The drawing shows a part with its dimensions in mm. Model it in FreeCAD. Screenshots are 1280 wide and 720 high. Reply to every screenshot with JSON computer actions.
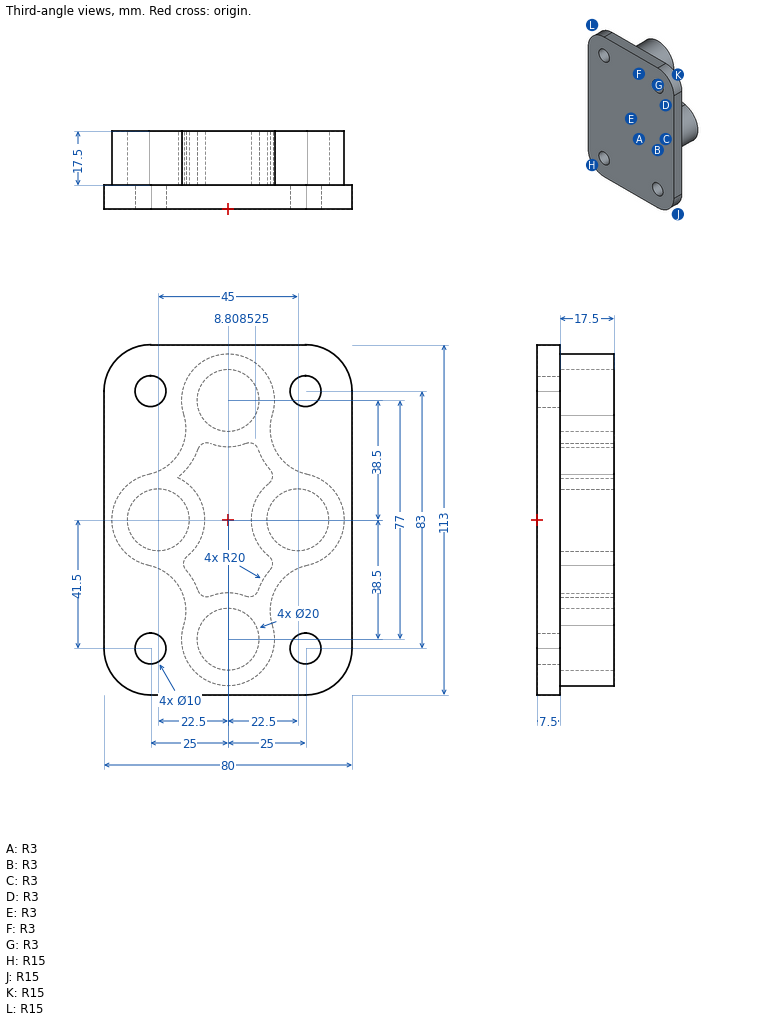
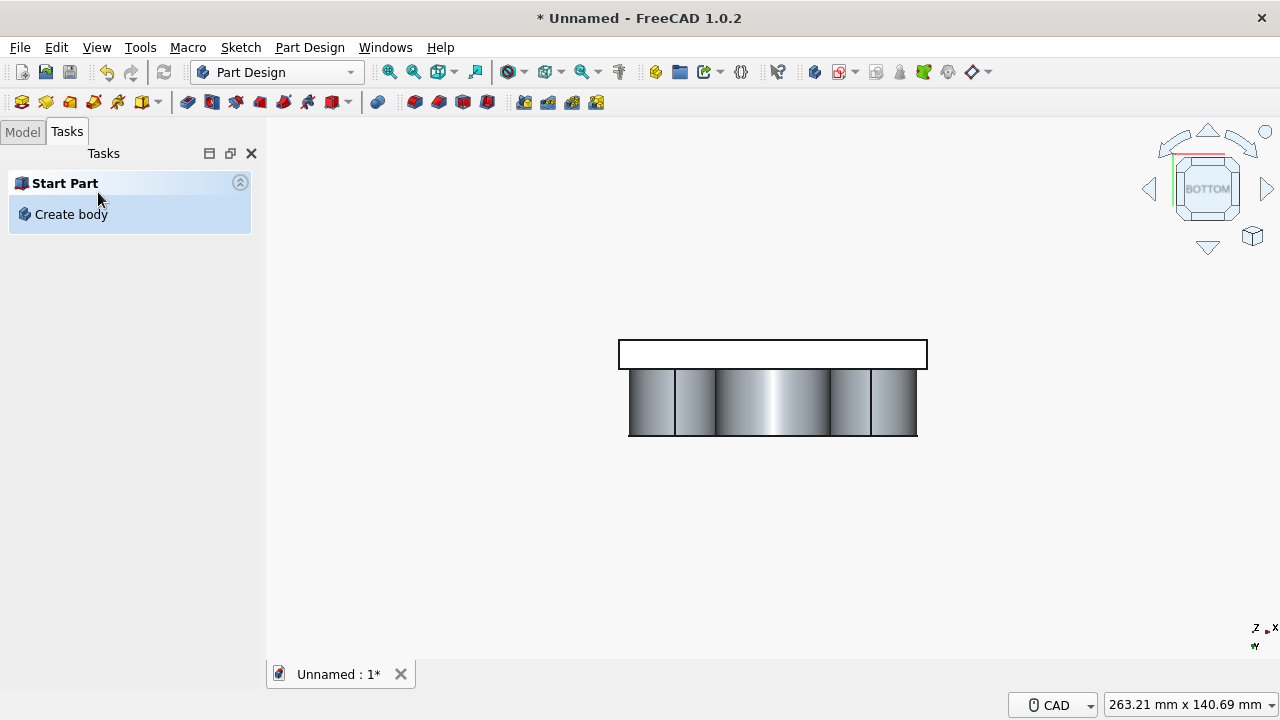
{"action": "key", "text": "4"}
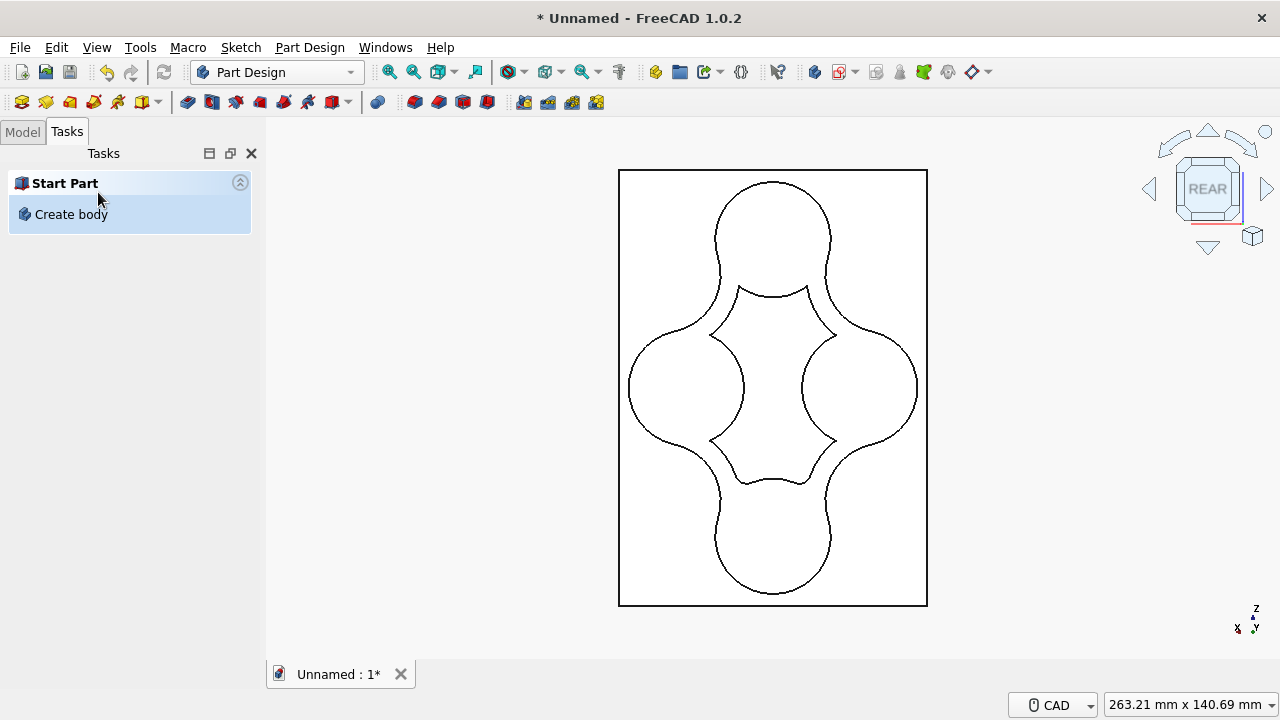
{"action": "key", "text": "6"}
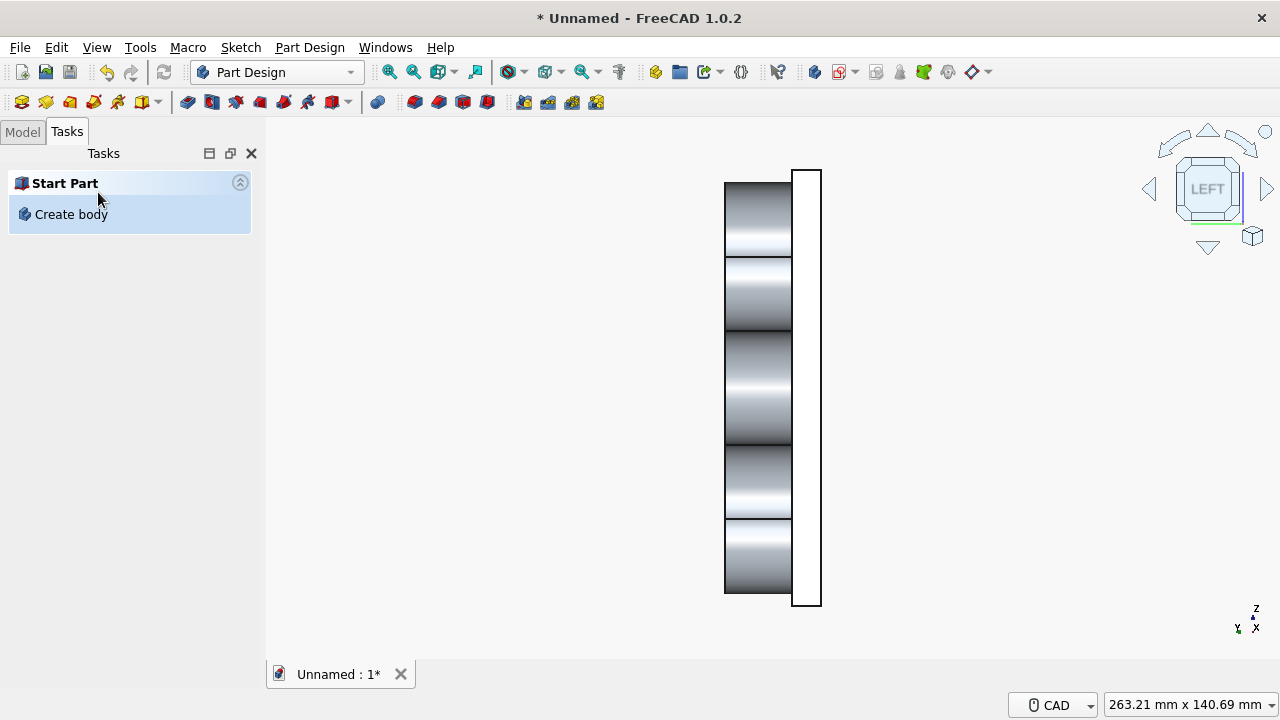
{"action": "key", "text": "v 3"}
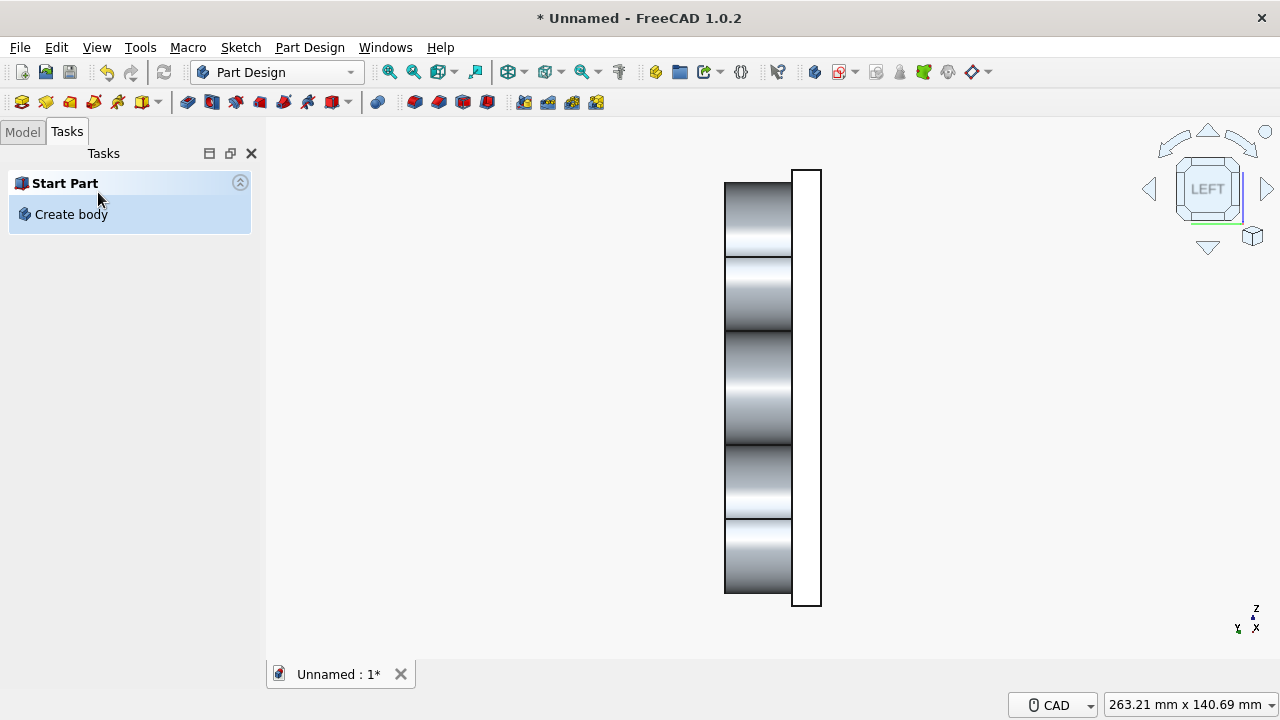
{"action": "key", "text": "0"}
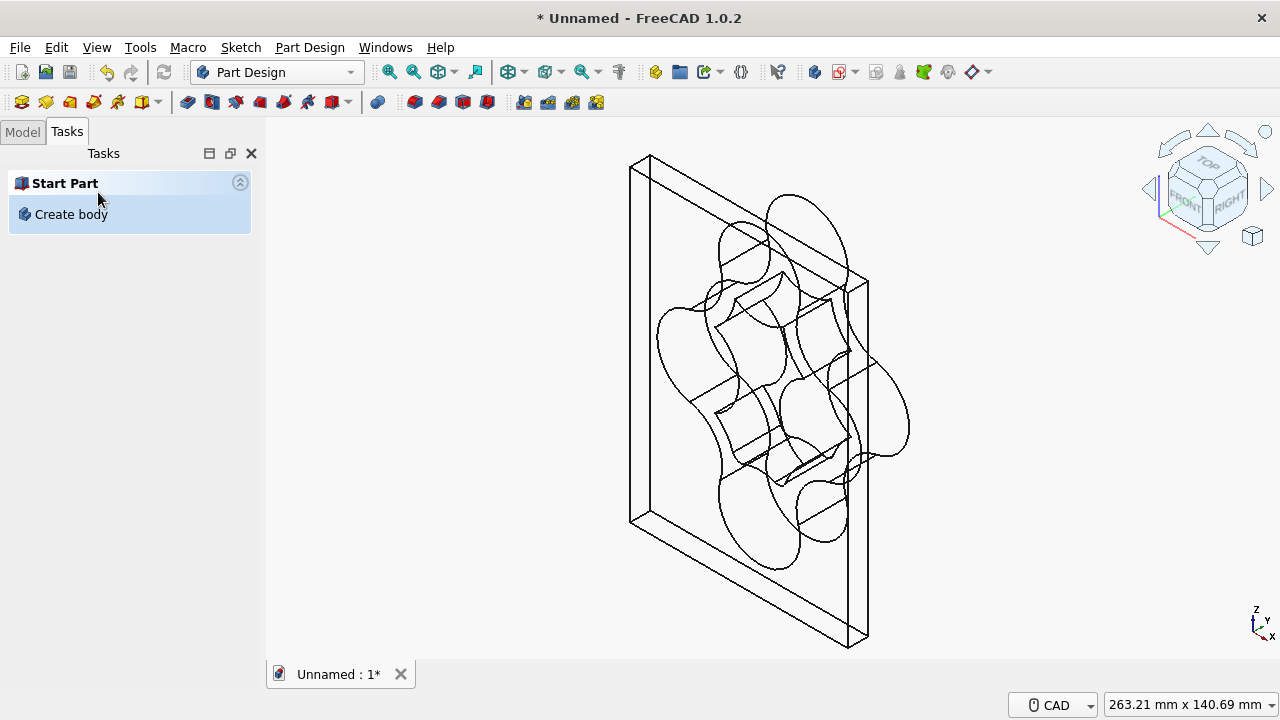
{"action": "left_click", "coordinate": [827, 450]}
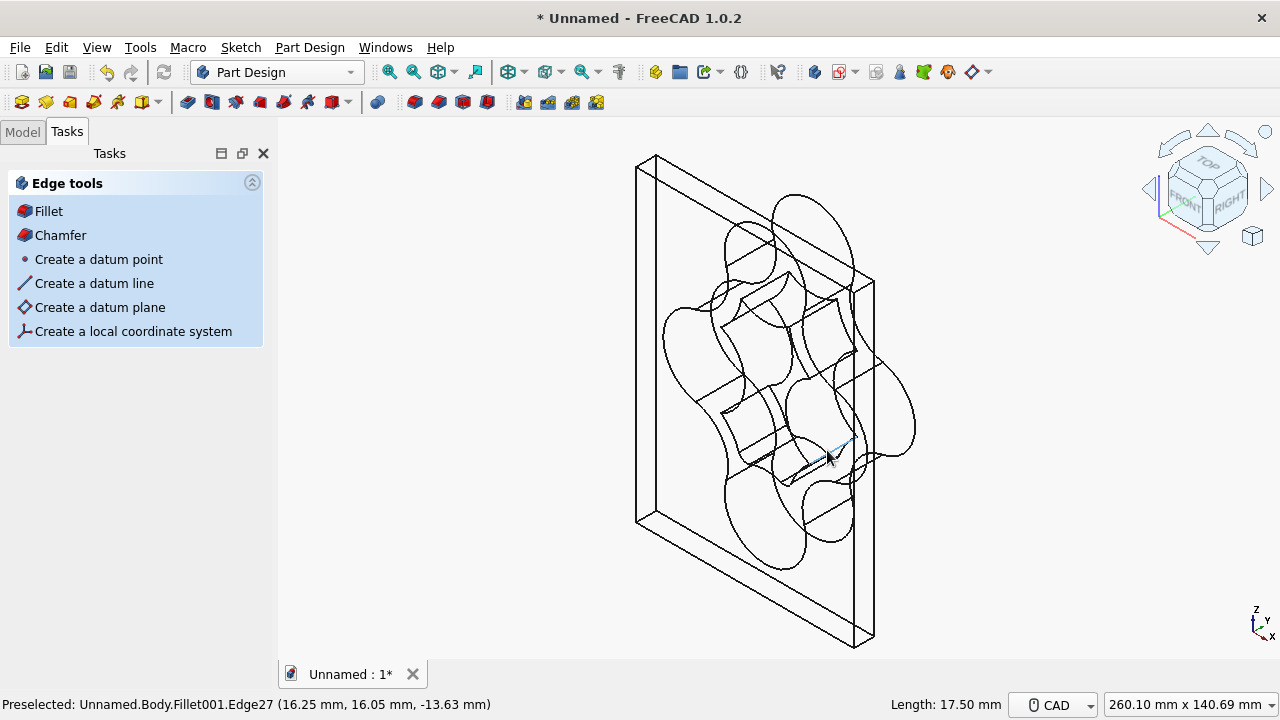
{"action": "key", "text": "v 1"}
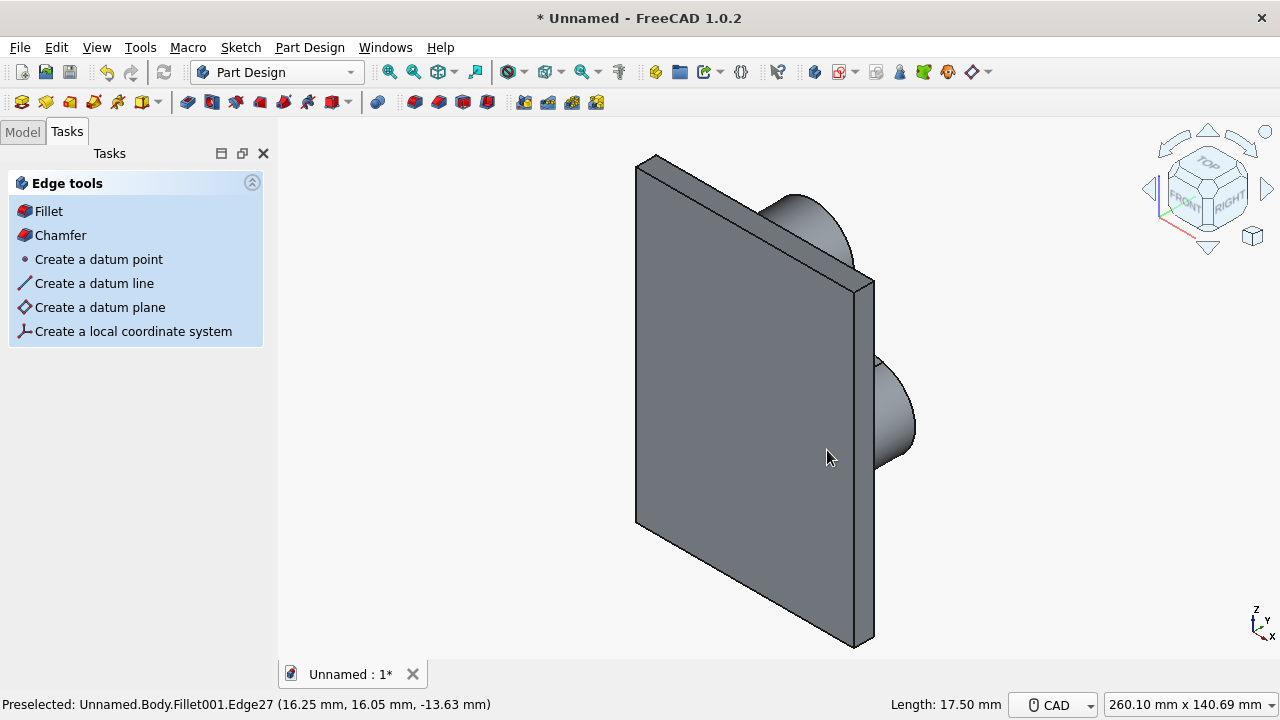
{"action": "left_click", "coordinate": [416, 102]}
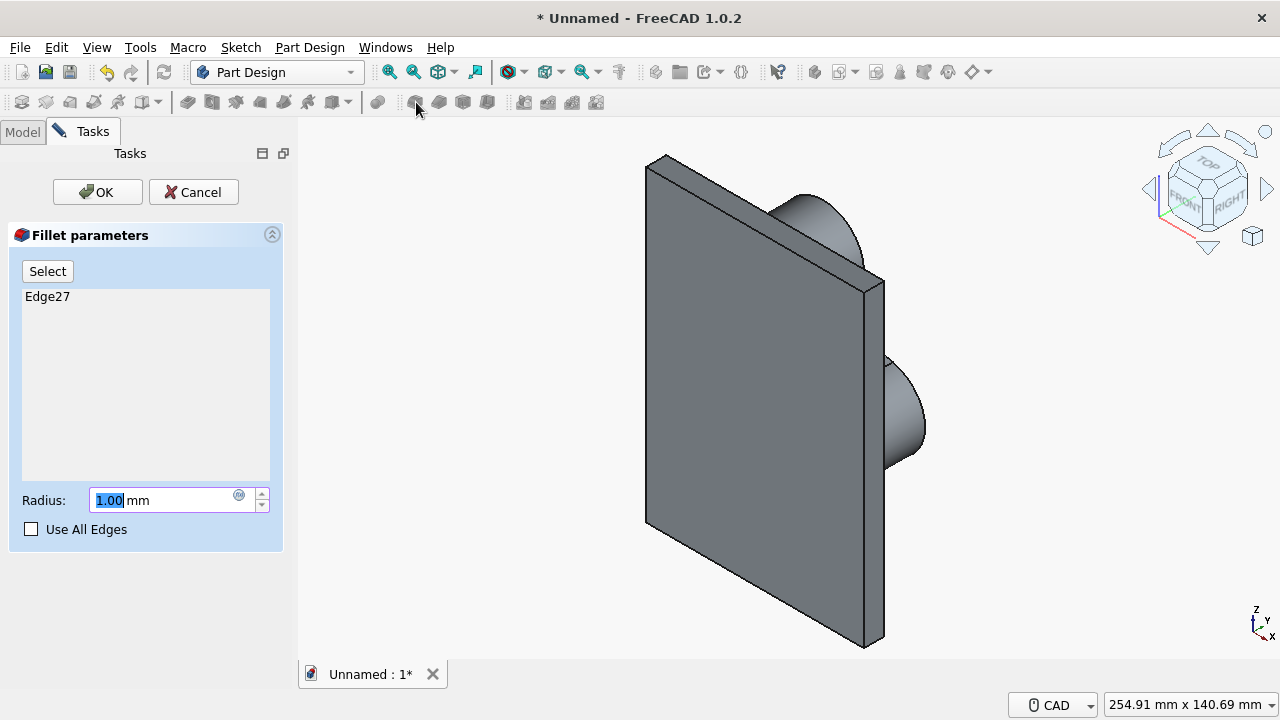
{"action": "type", "text": "3"}
{"action": "key", "text": "Tab"}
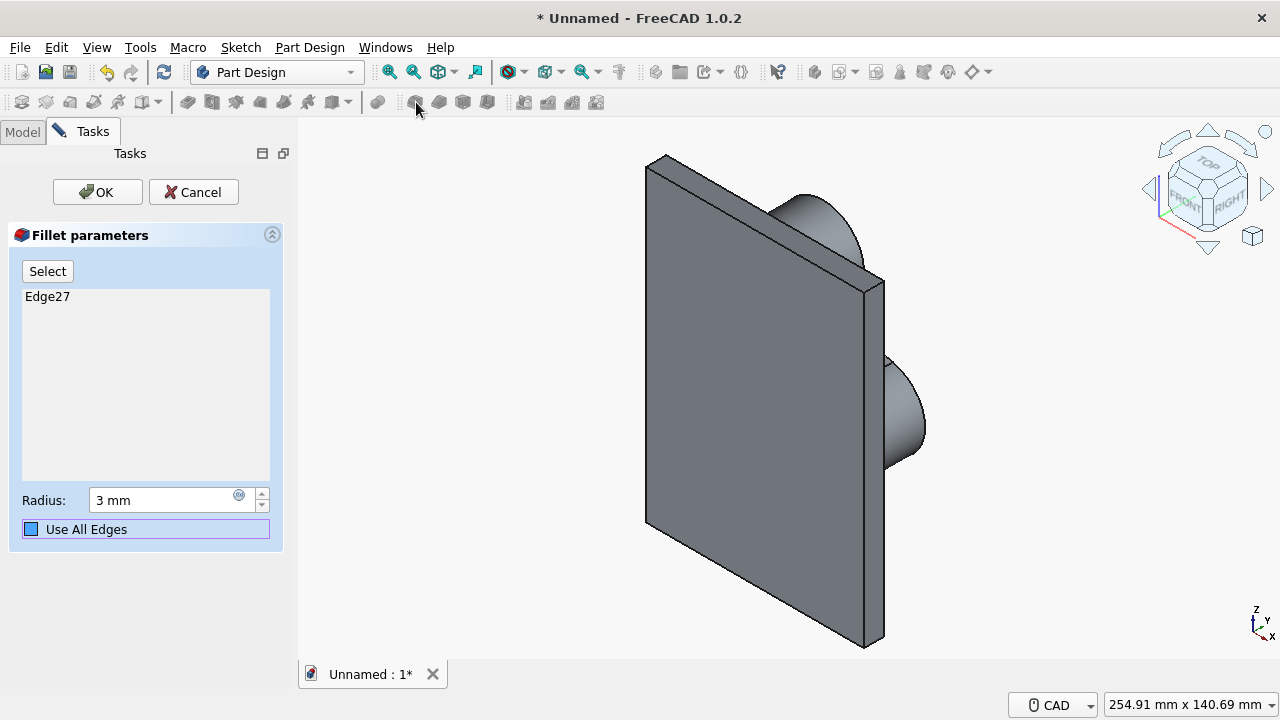
{"action": "left_click", "coordinate": [98, 192]}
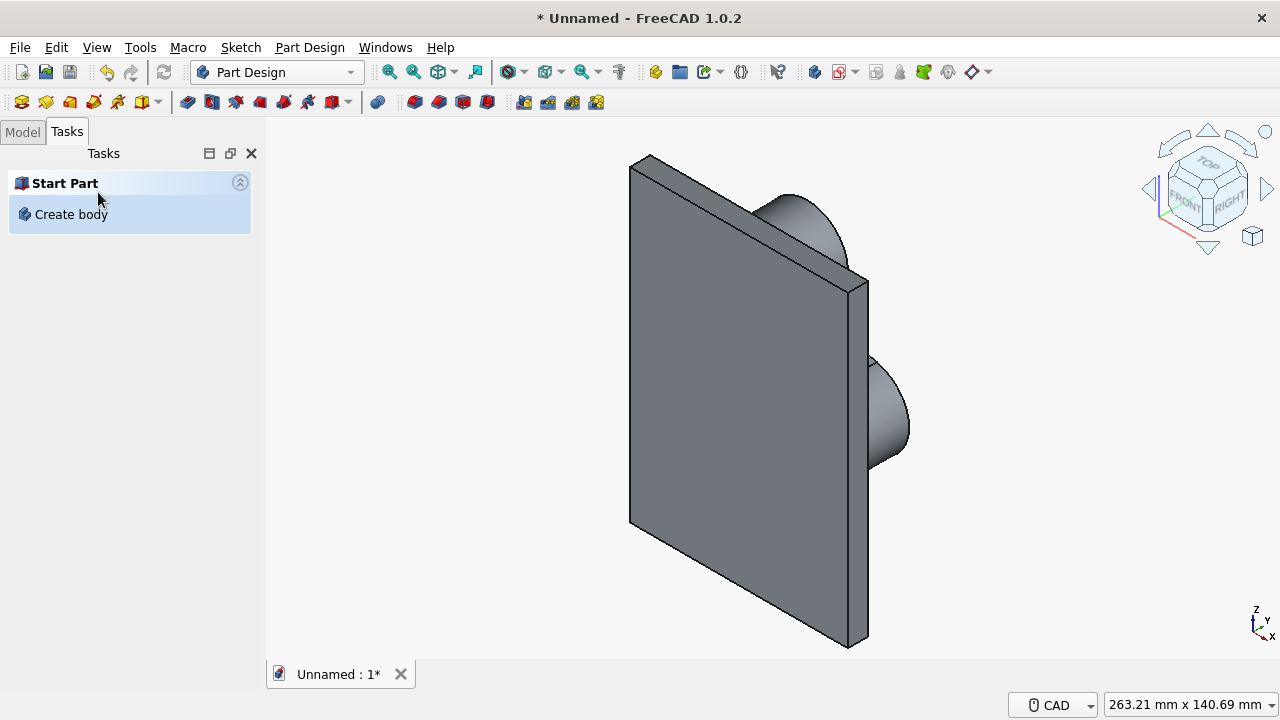
{"action": "key", "text": "2"}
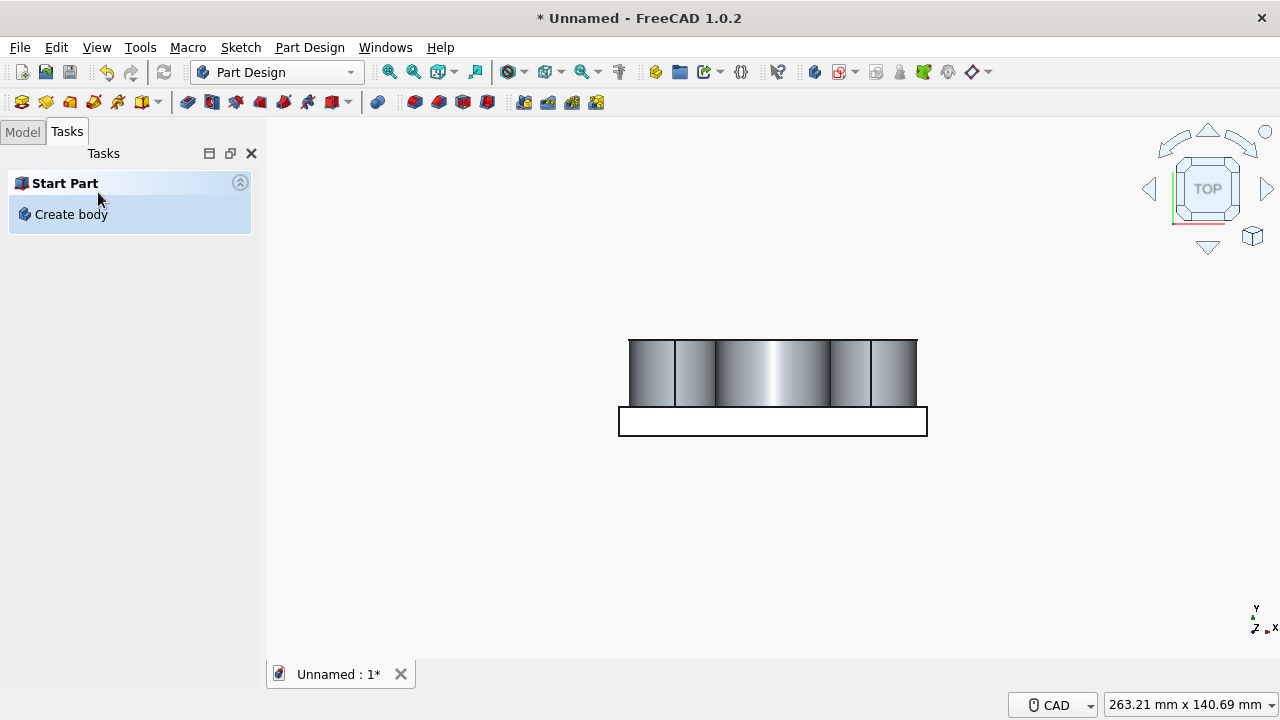
{"action": "key", "text": "v f"}